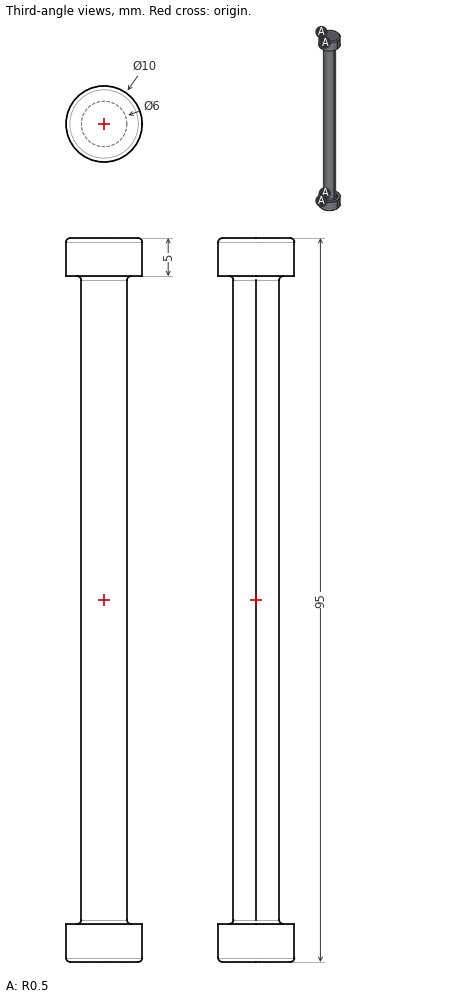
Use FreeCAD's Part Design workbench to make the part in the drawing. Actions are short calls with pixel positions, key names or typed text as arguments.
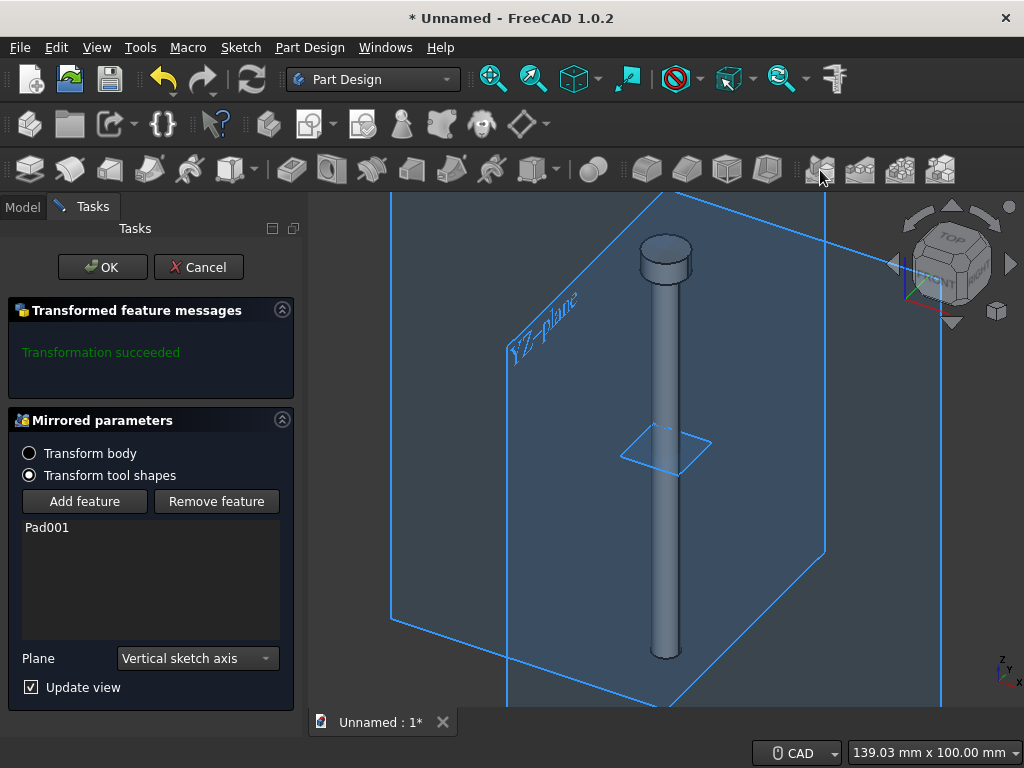
click(198, 658)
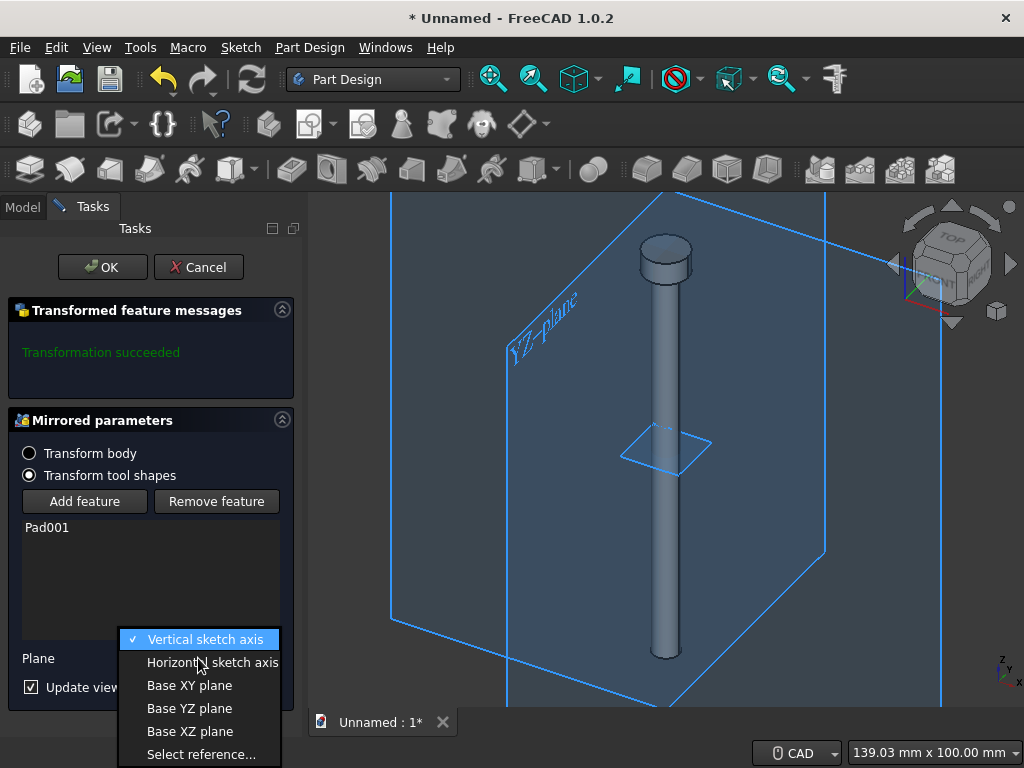
click(198, 686)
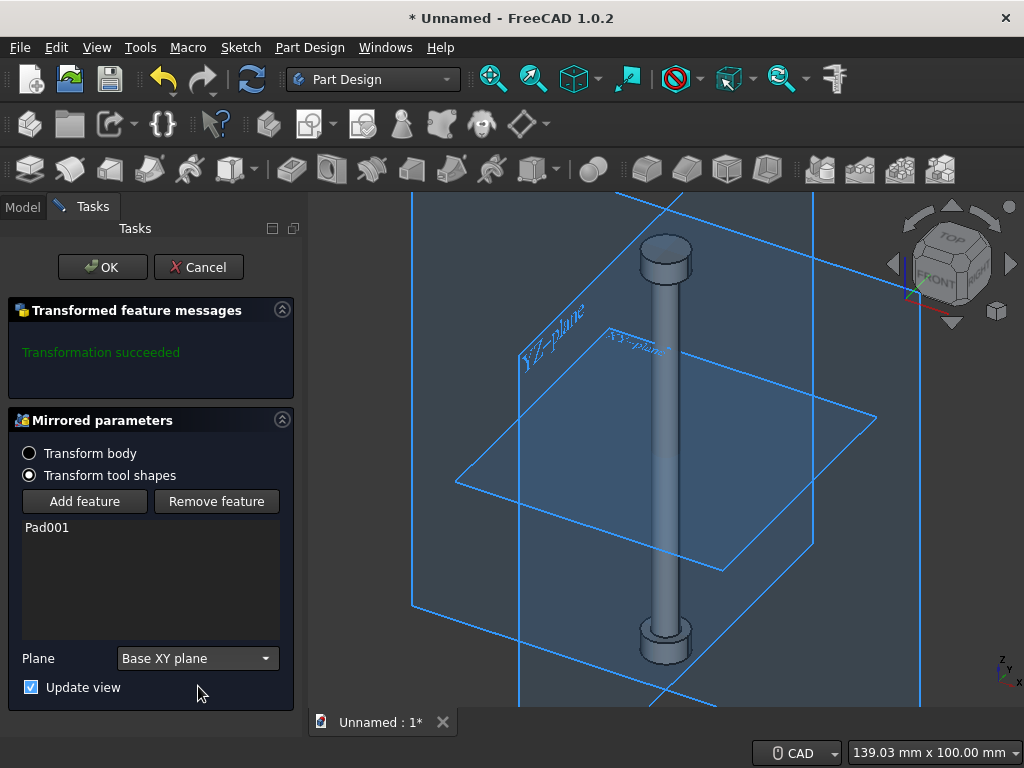
click(103, 267)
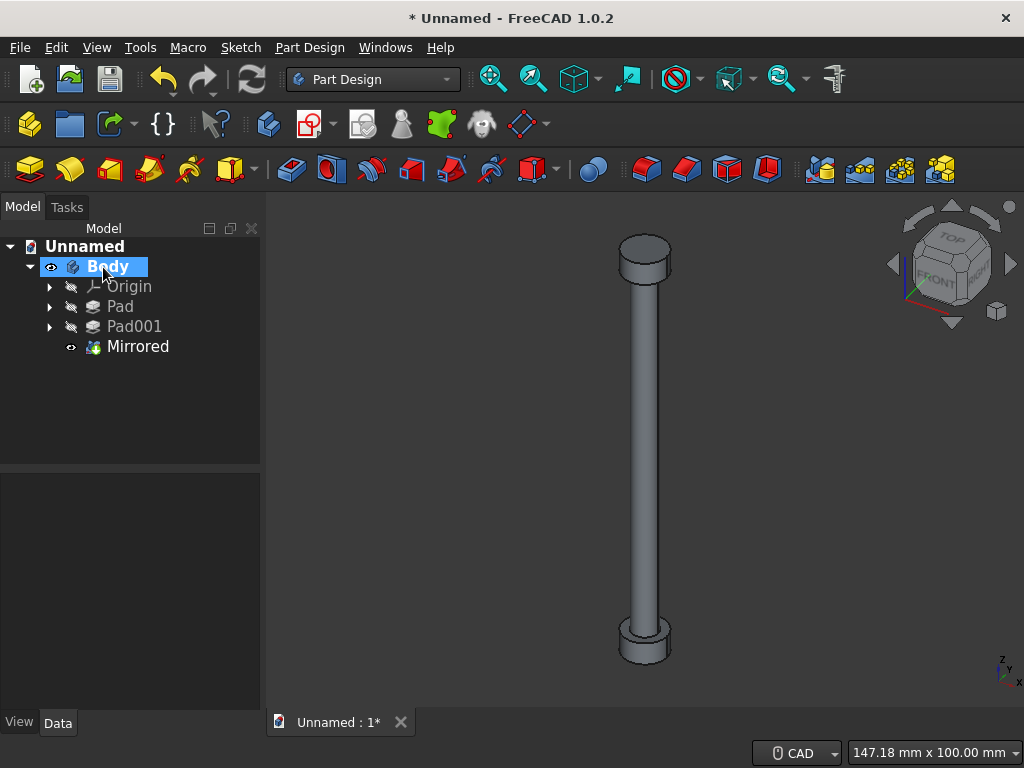
click(619, 250)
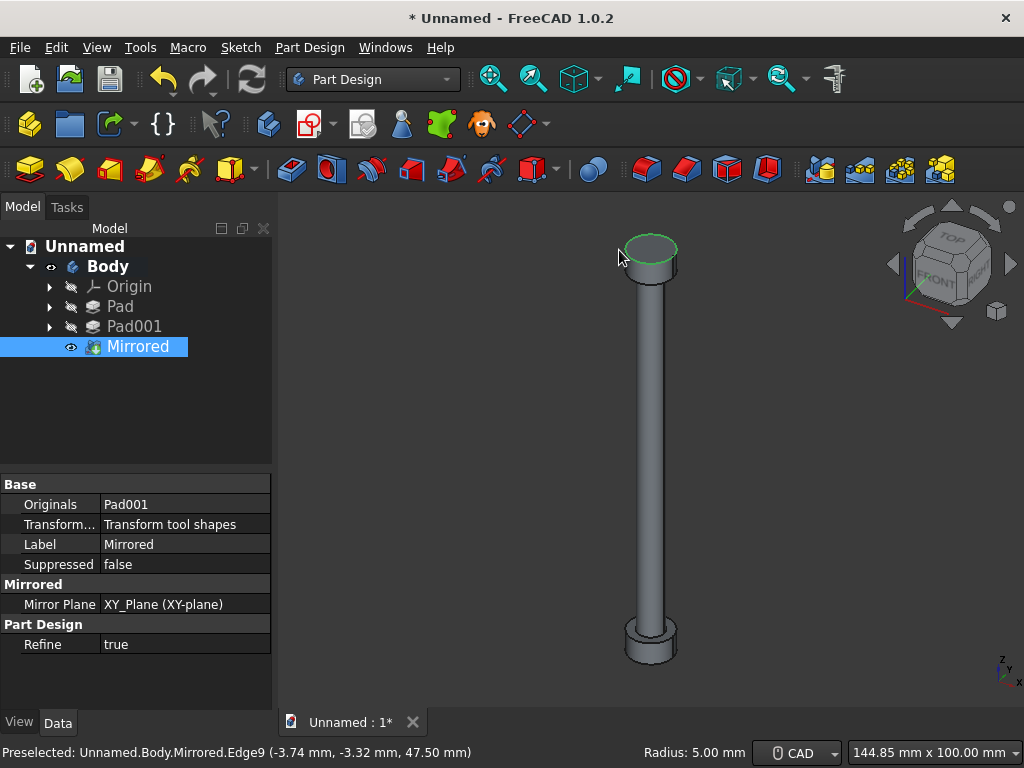
key(0)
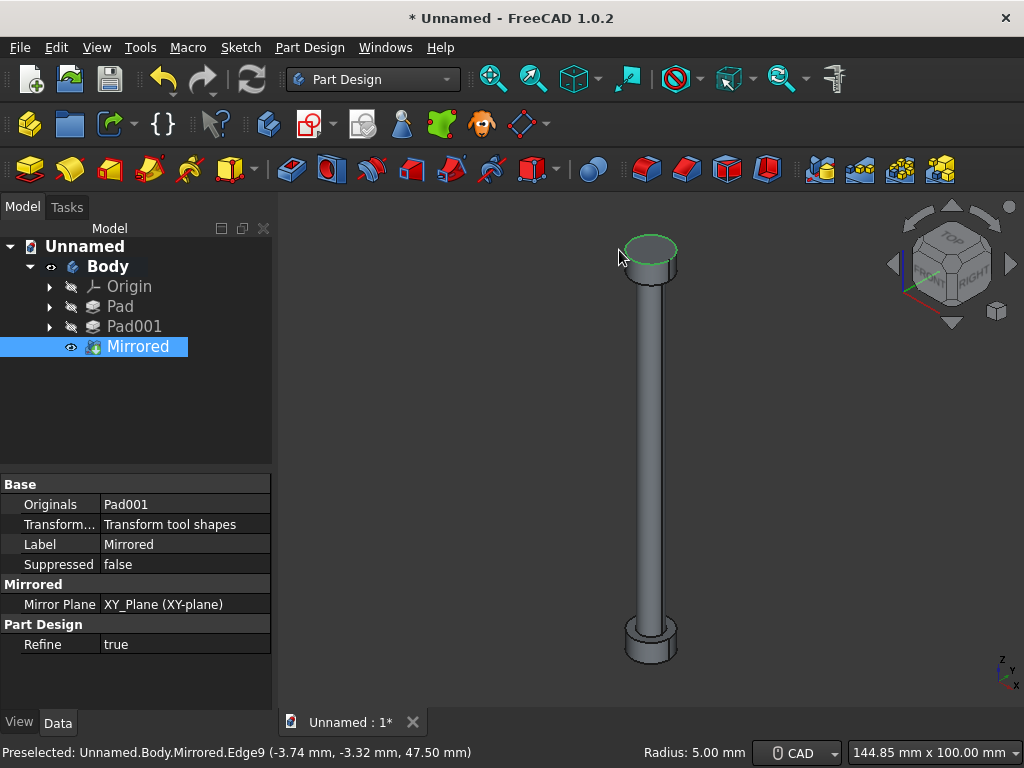
click(628, 655, ctrl)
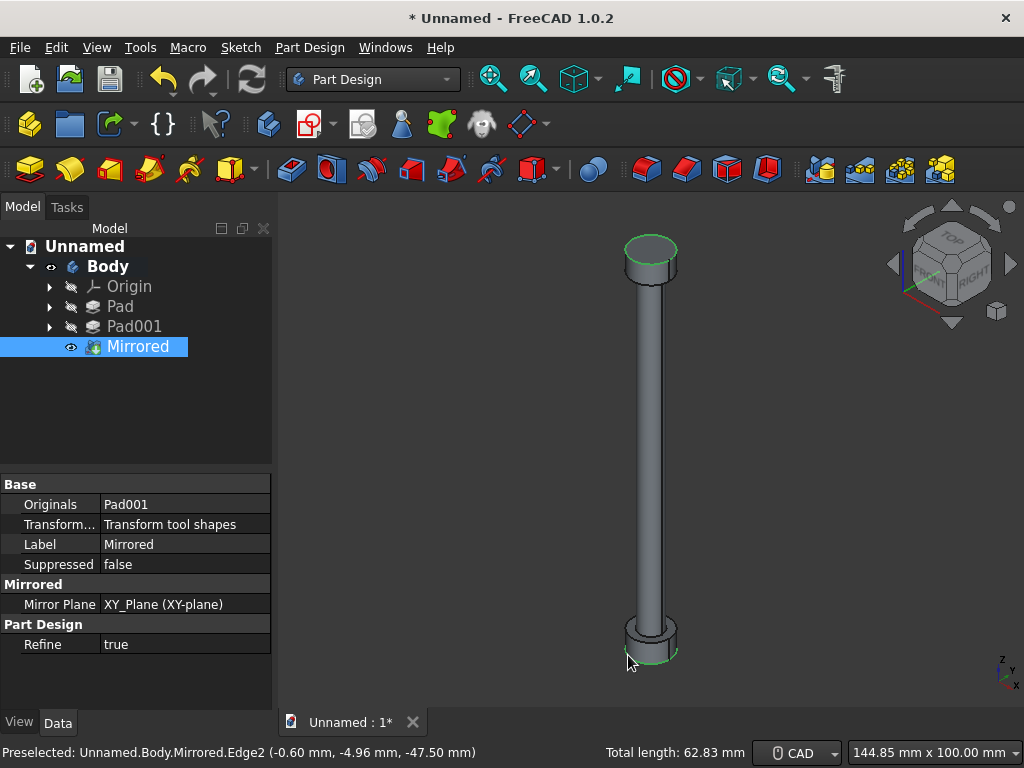
key(2)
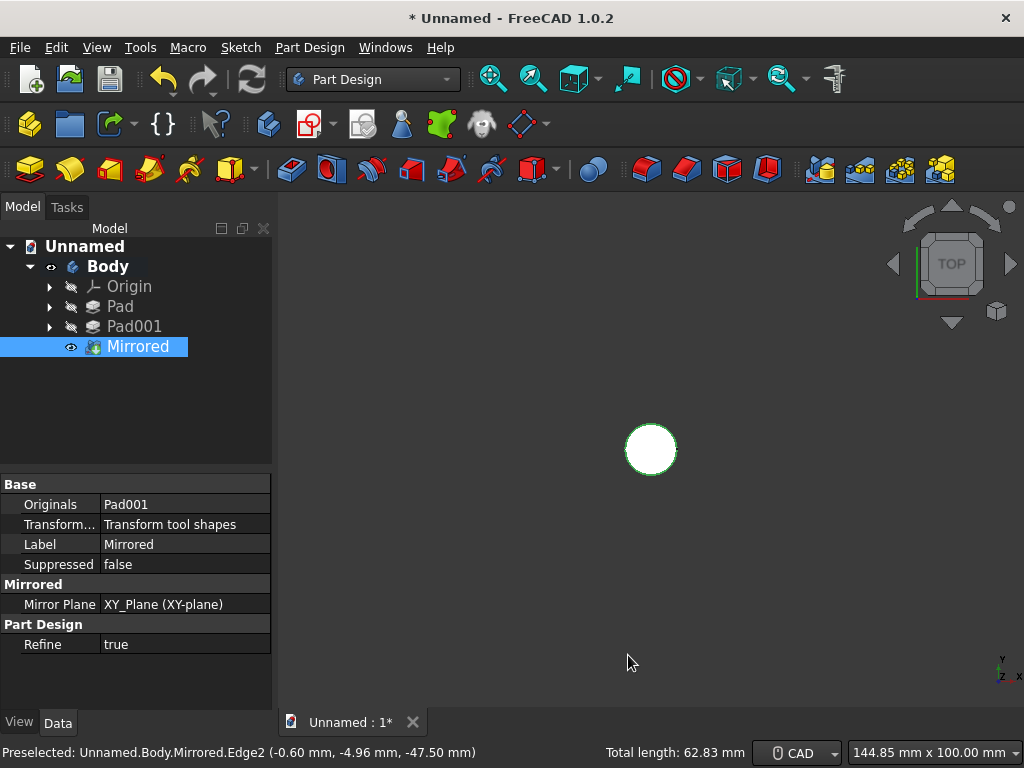
click(494, 80)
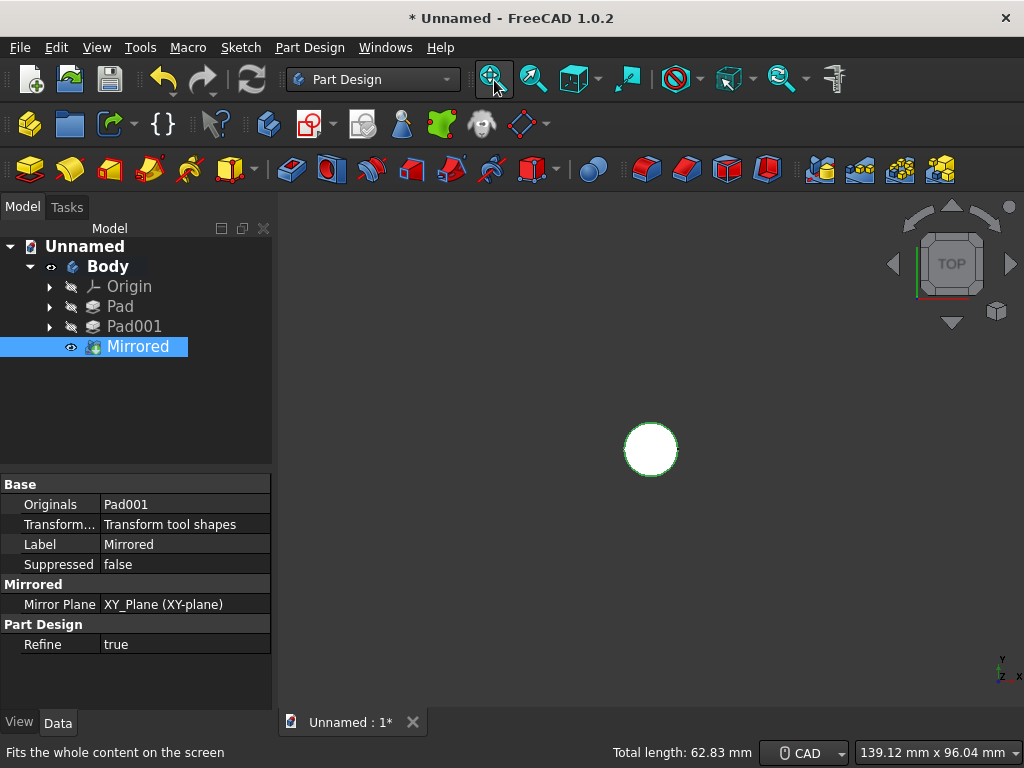
key(1)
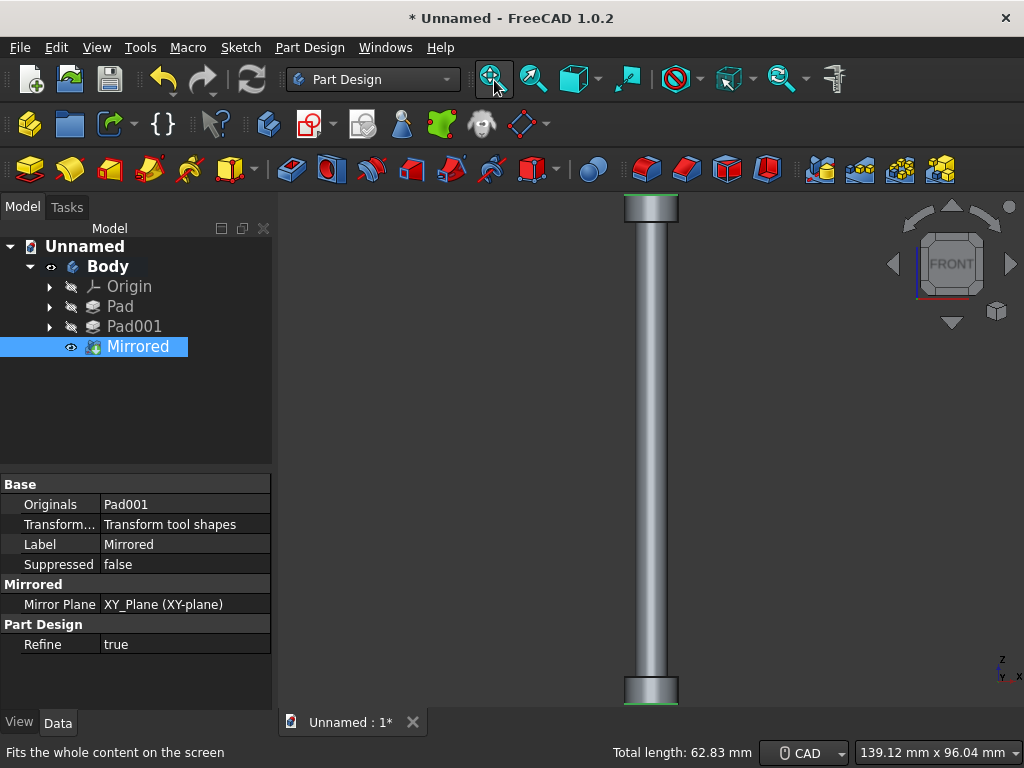
key(3)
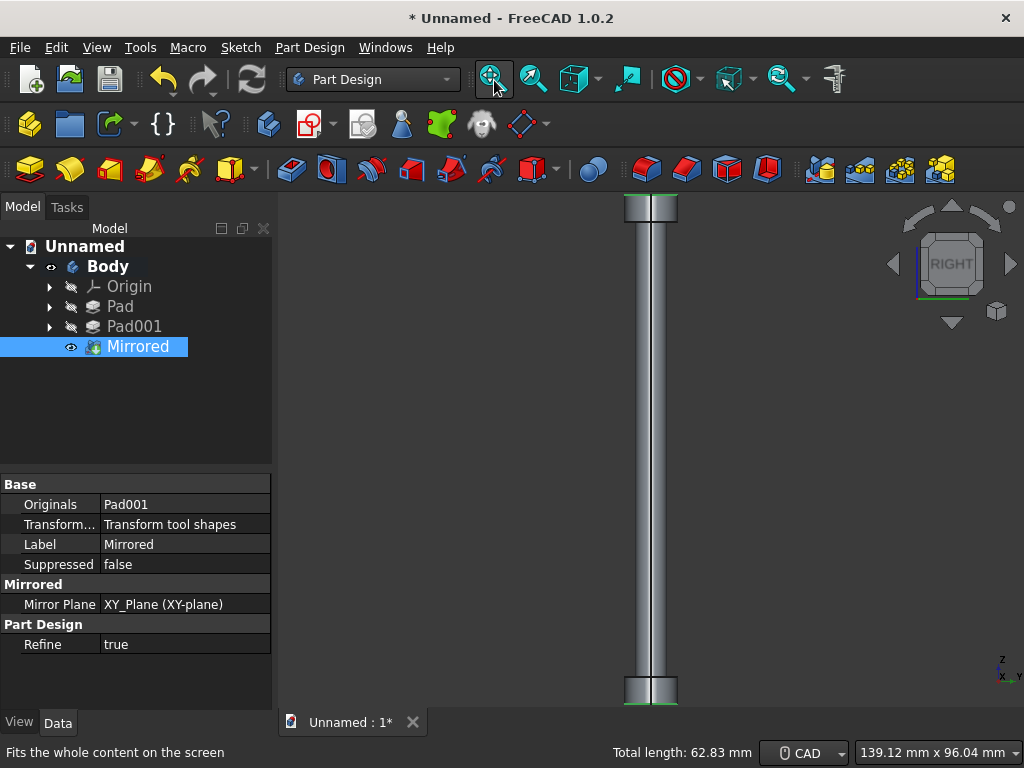
key(5)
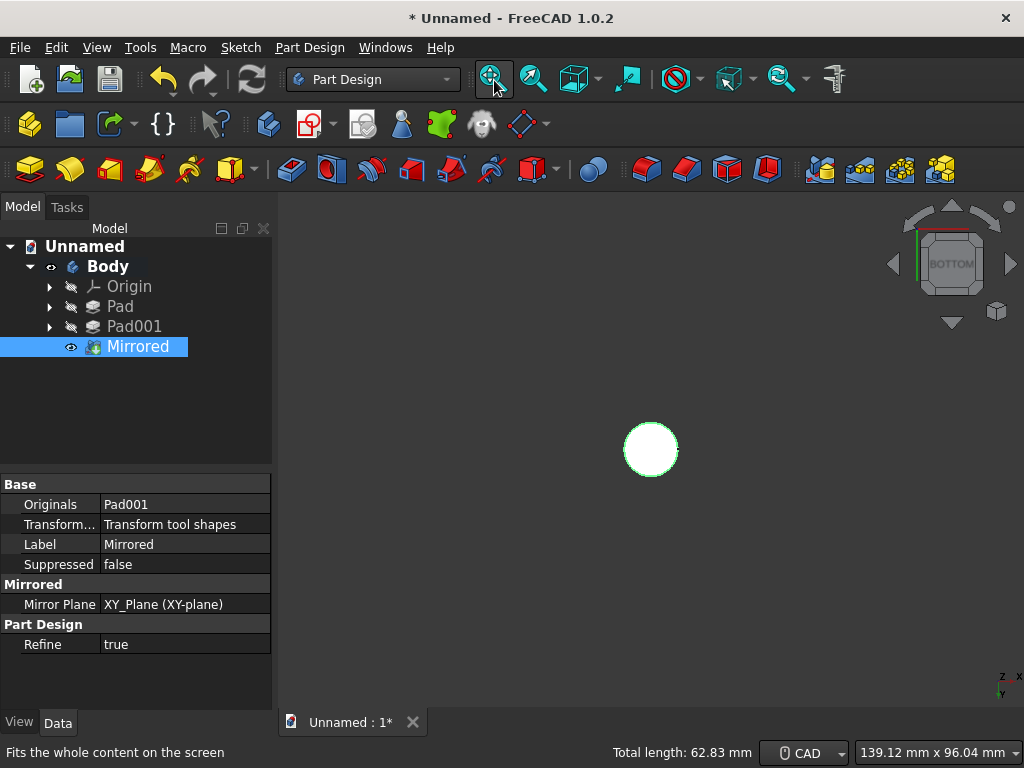
click(494, 80)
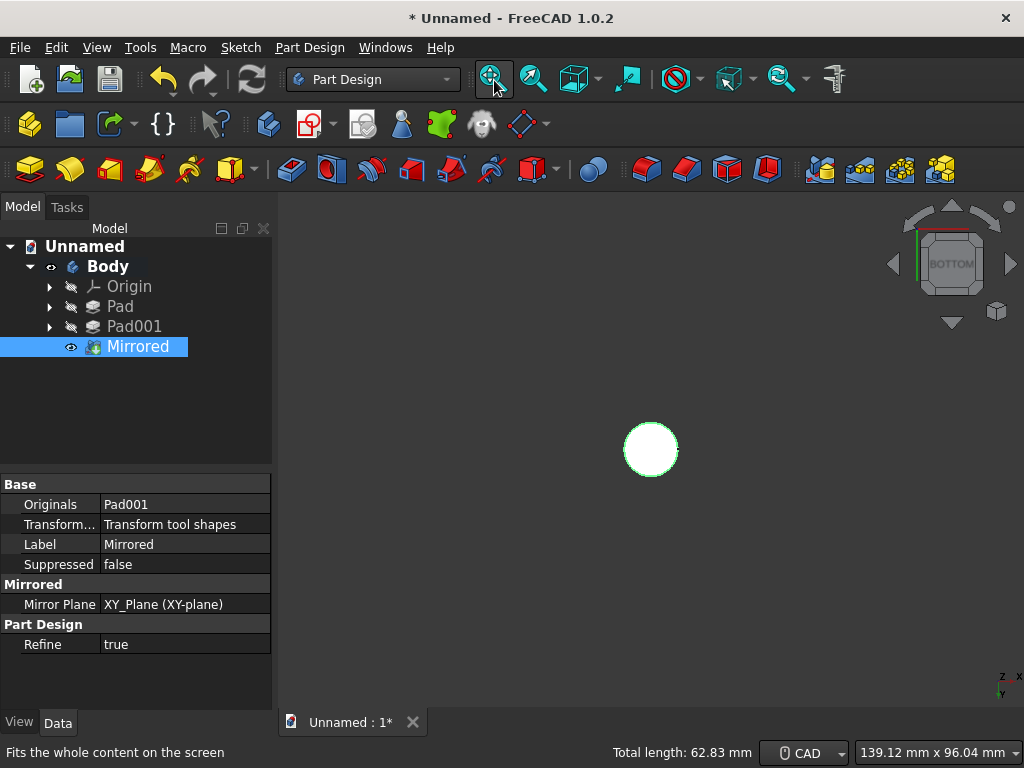
key(4)